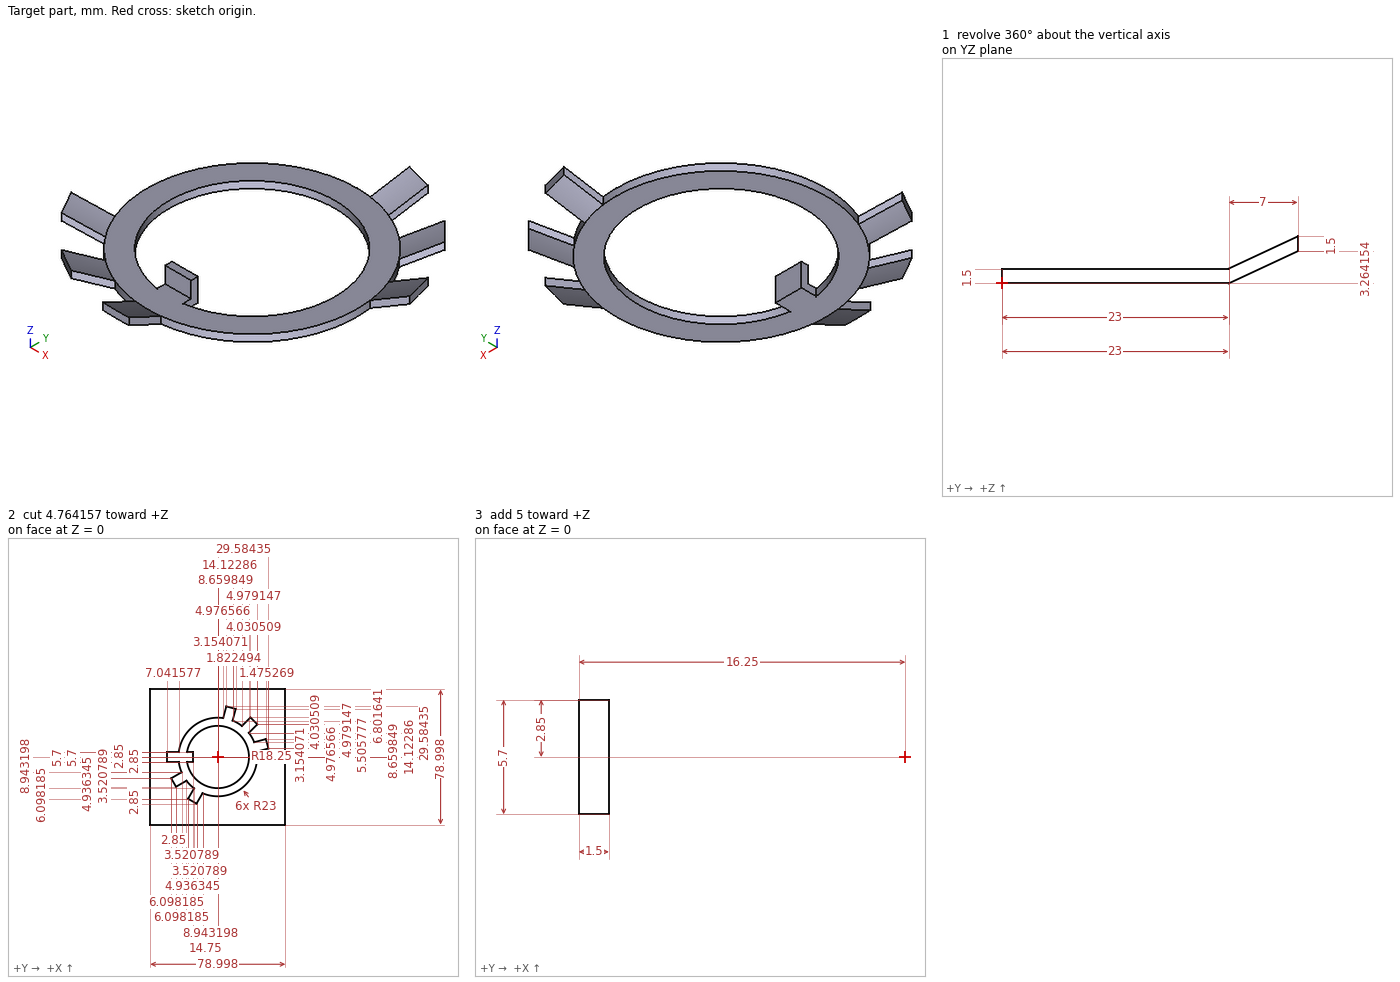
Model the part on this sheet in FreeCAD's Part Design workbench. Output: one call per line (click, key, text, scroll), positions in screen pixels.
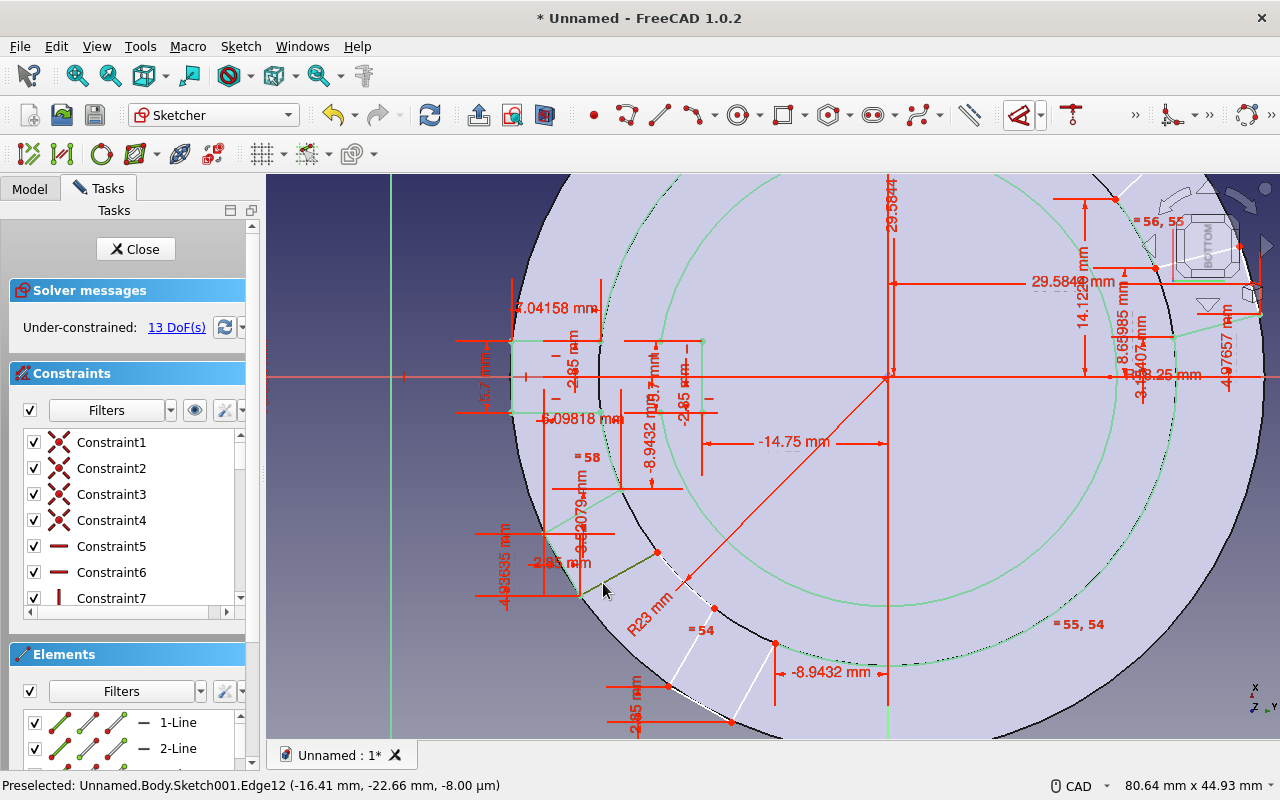
key(l)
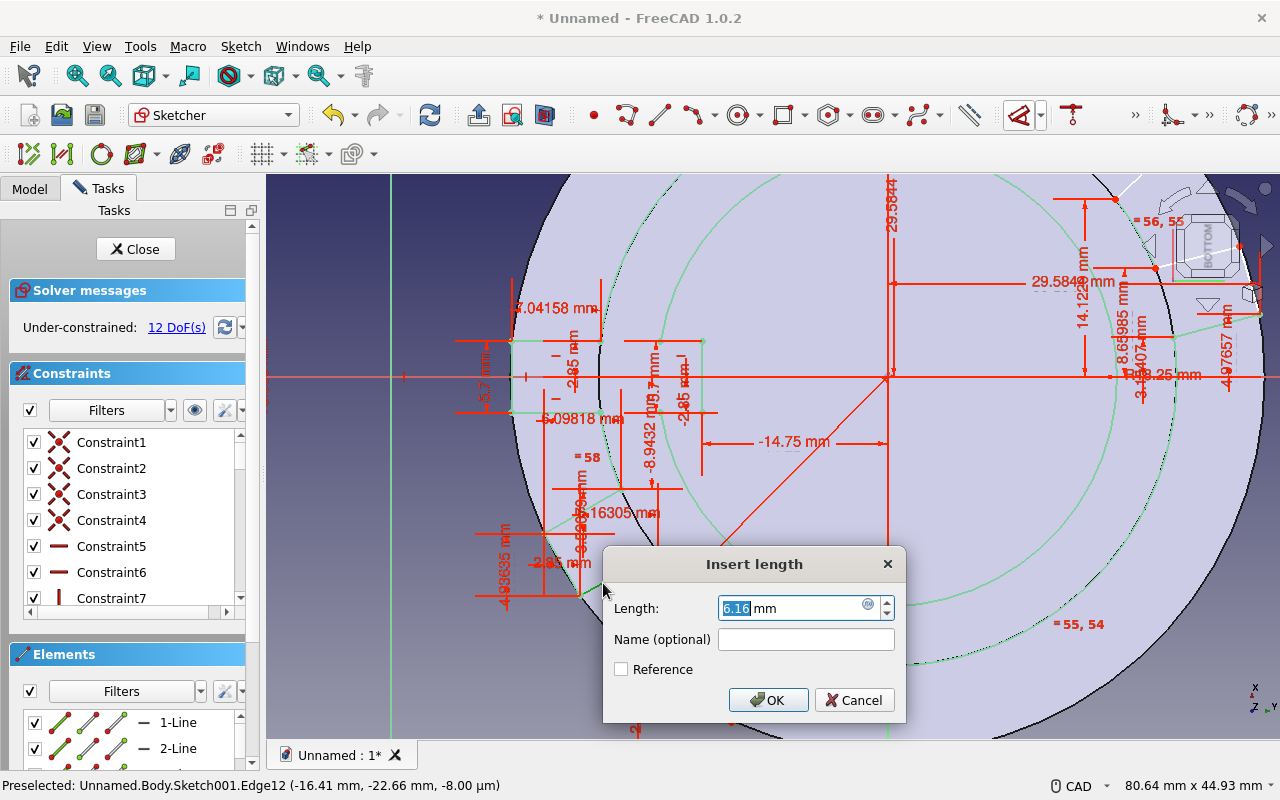
text(6.098185)
key(Return)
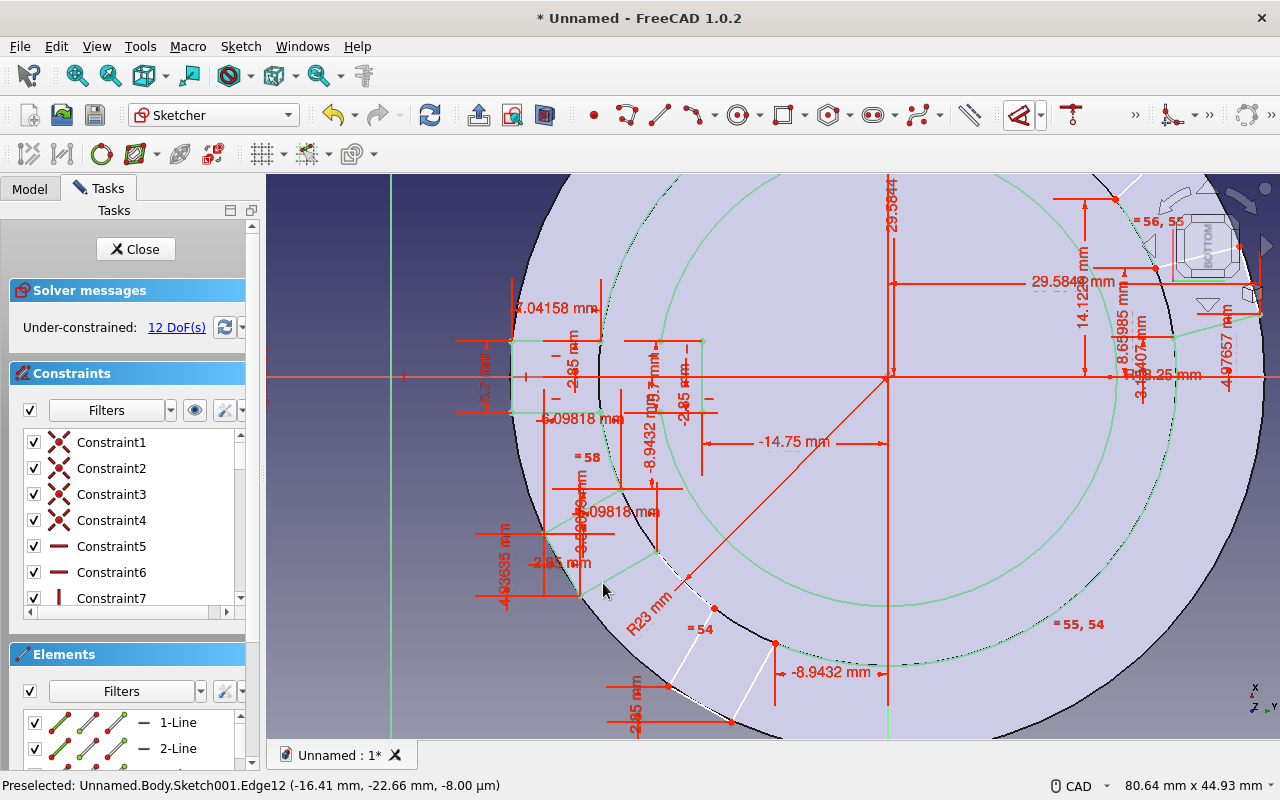
click(683, 663)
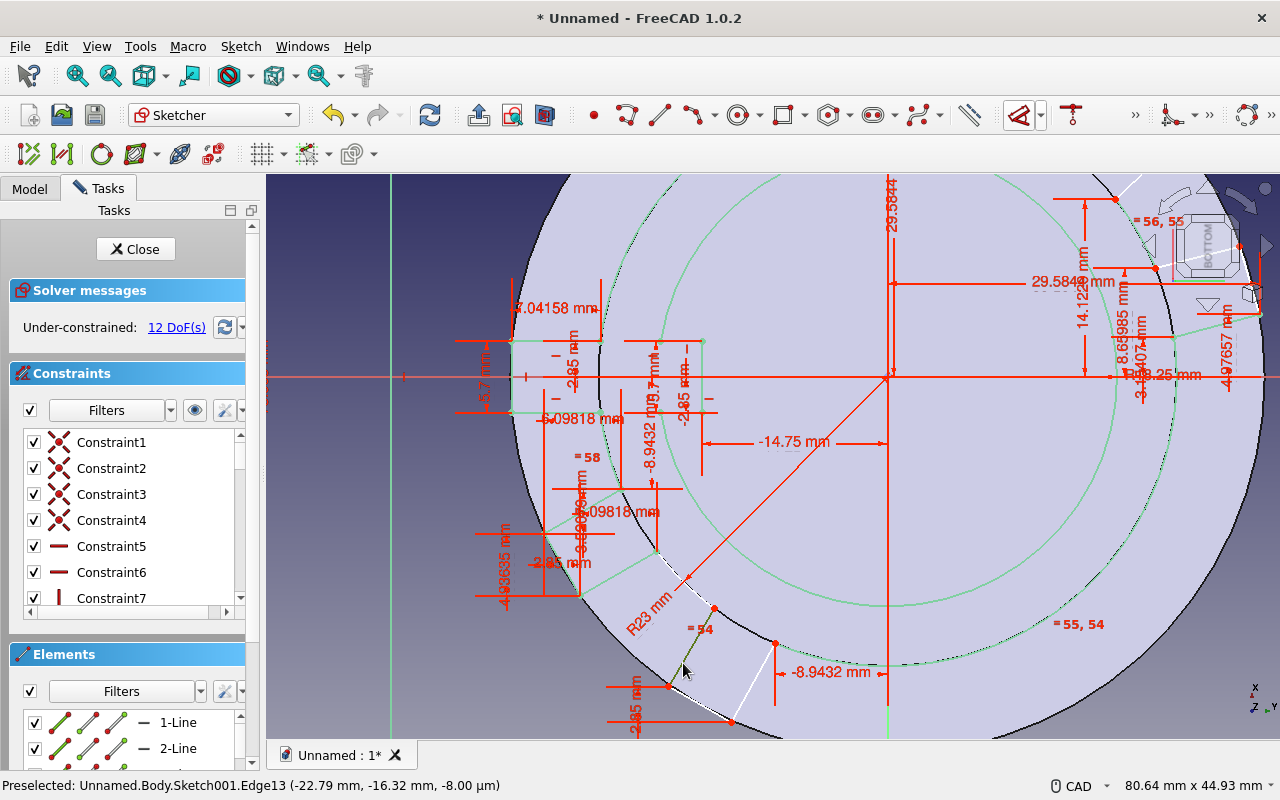
key(l)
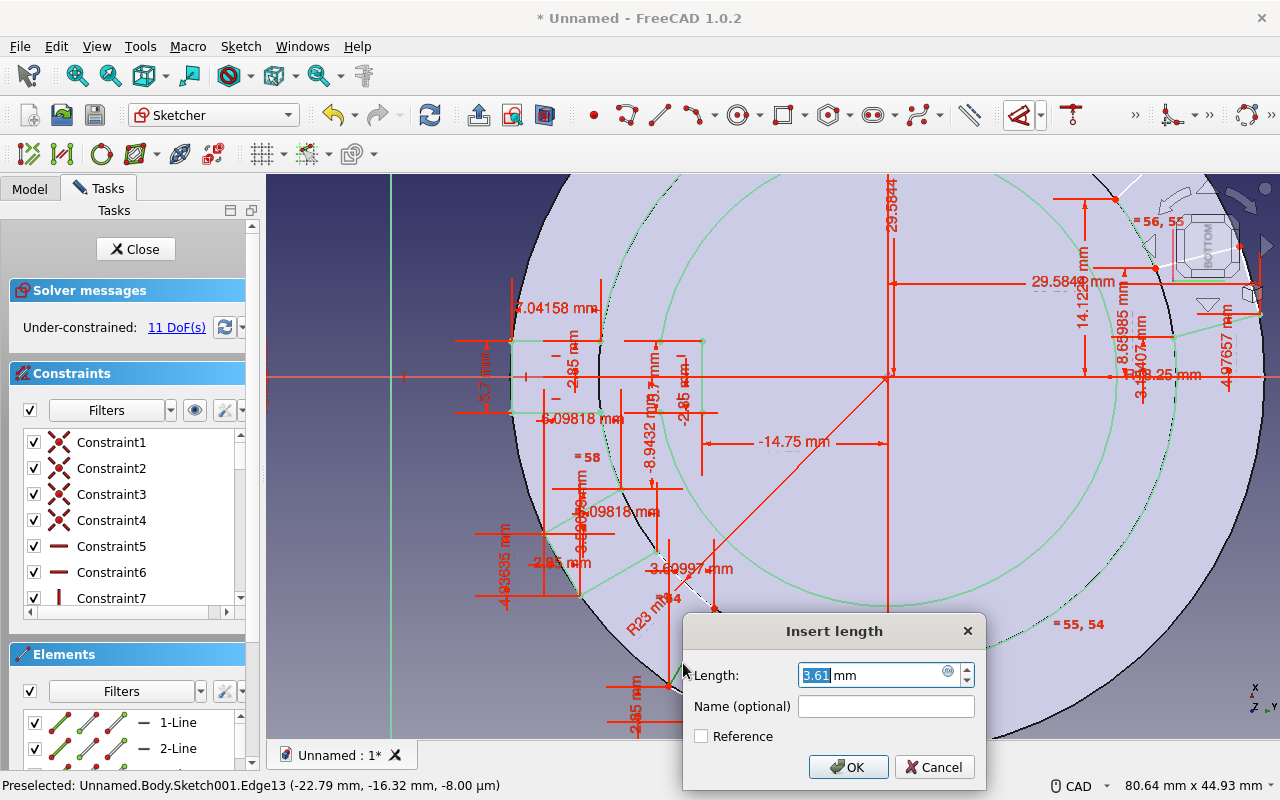
text(3.520789)
key(Return)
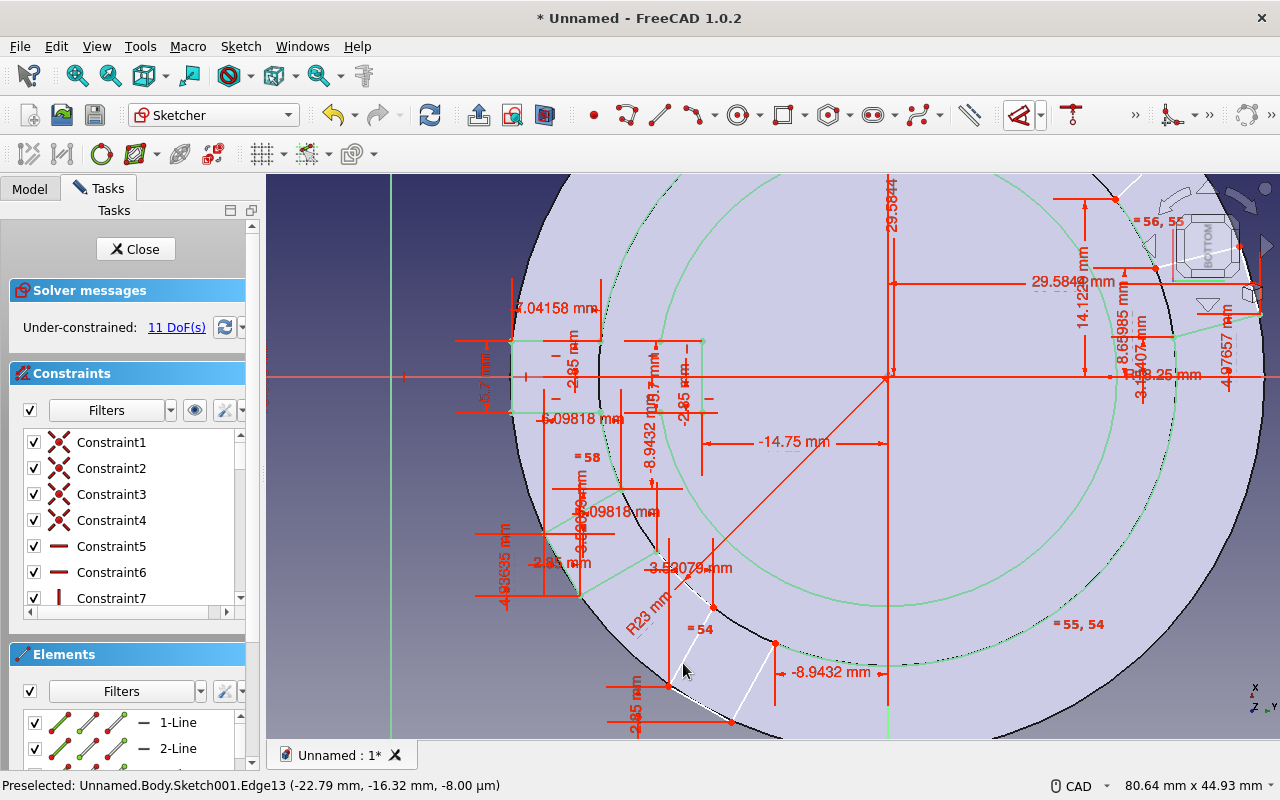
click(682, 663)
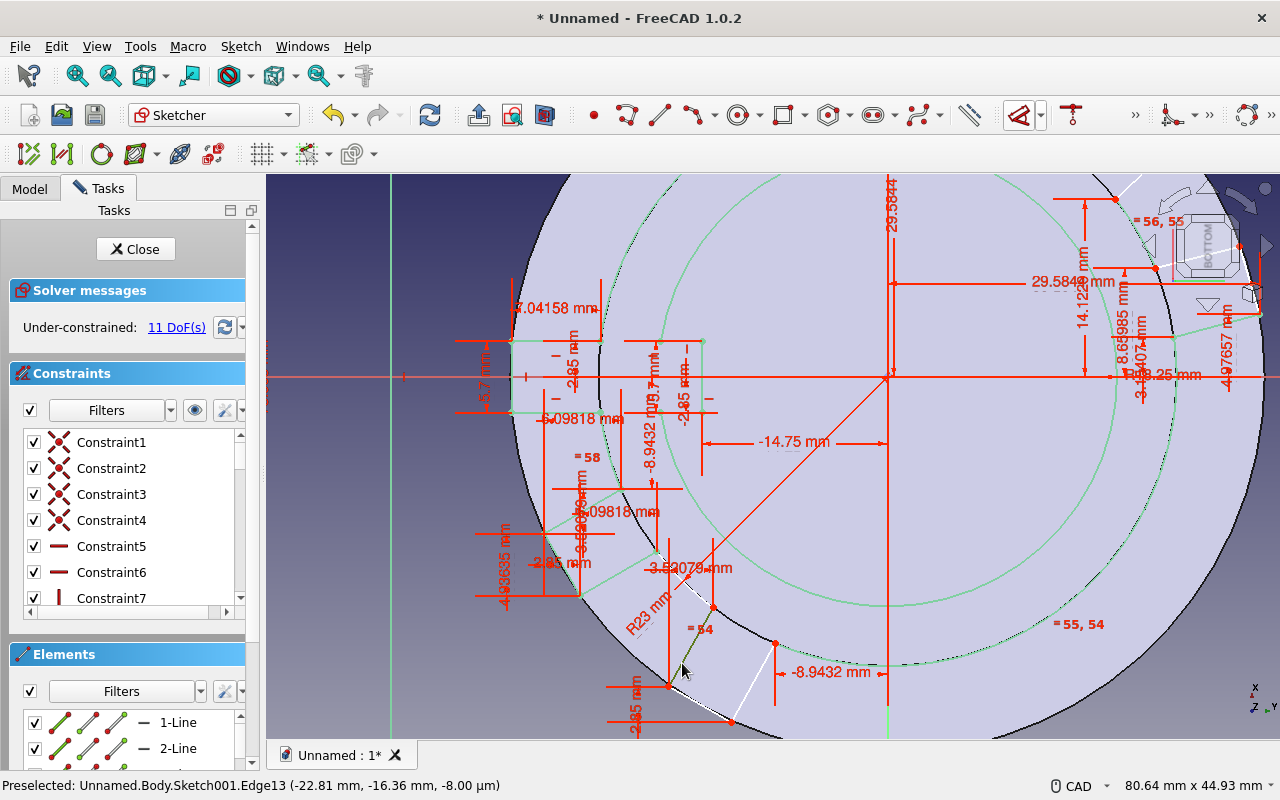
click(1040, 116)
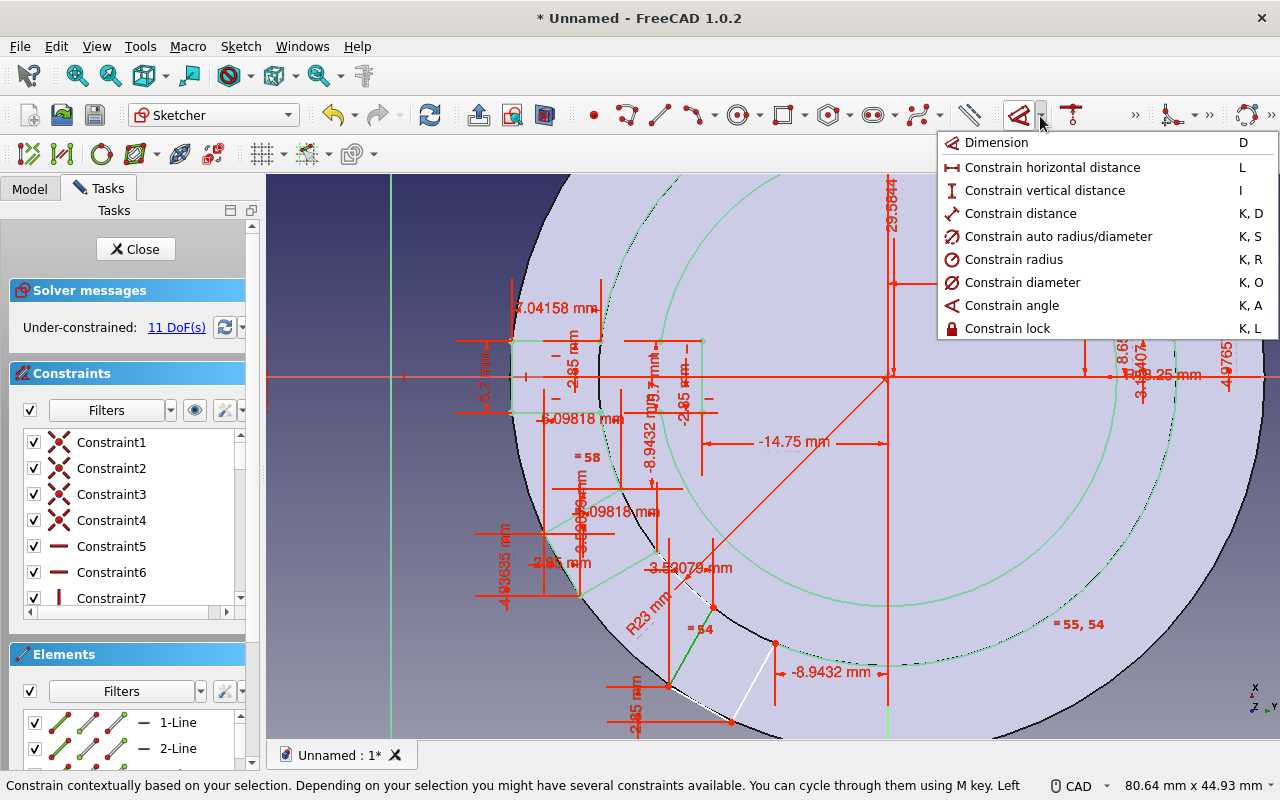
click(1108, 190)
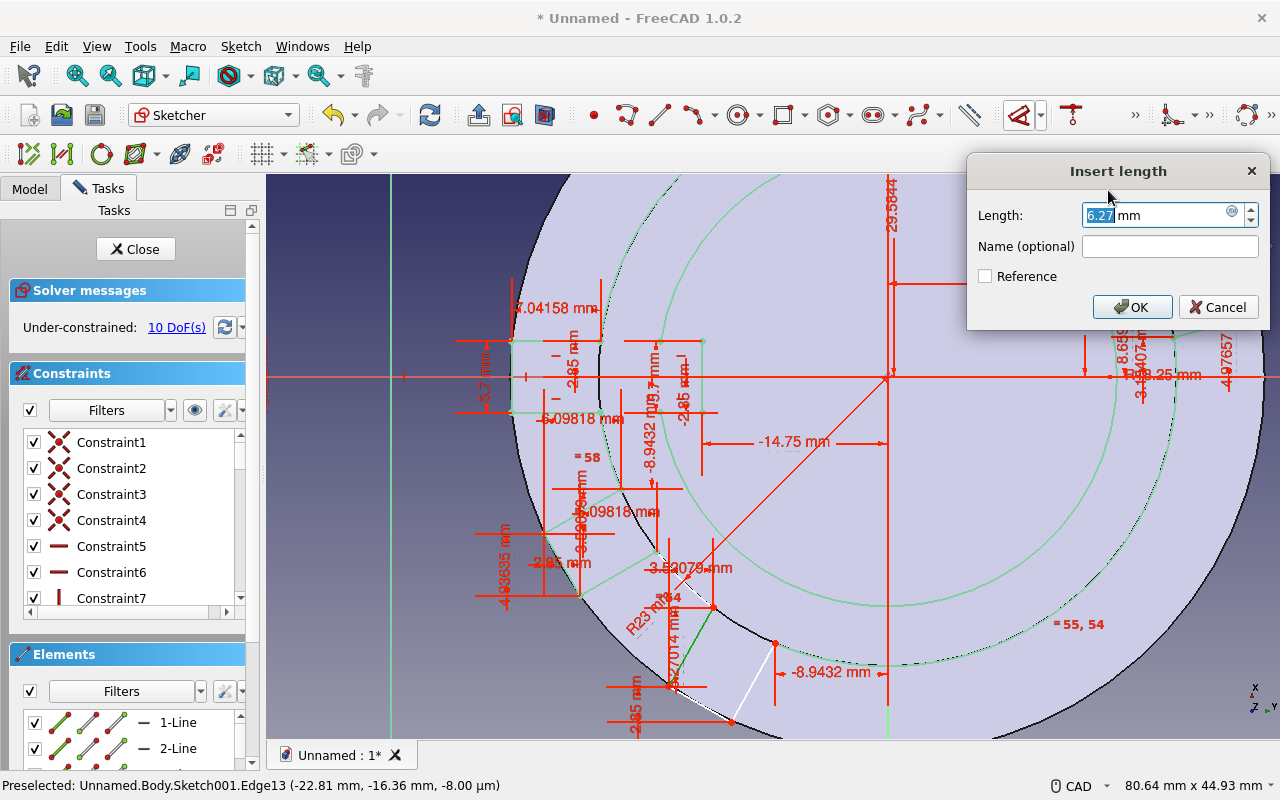
text(6.098185)
key(Return)